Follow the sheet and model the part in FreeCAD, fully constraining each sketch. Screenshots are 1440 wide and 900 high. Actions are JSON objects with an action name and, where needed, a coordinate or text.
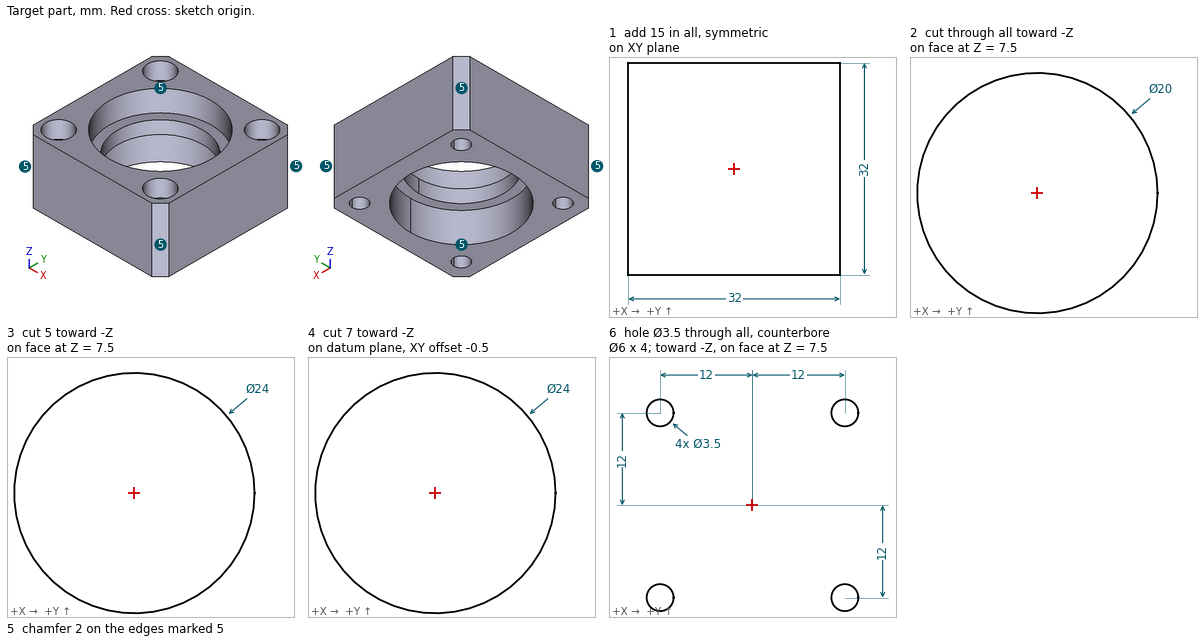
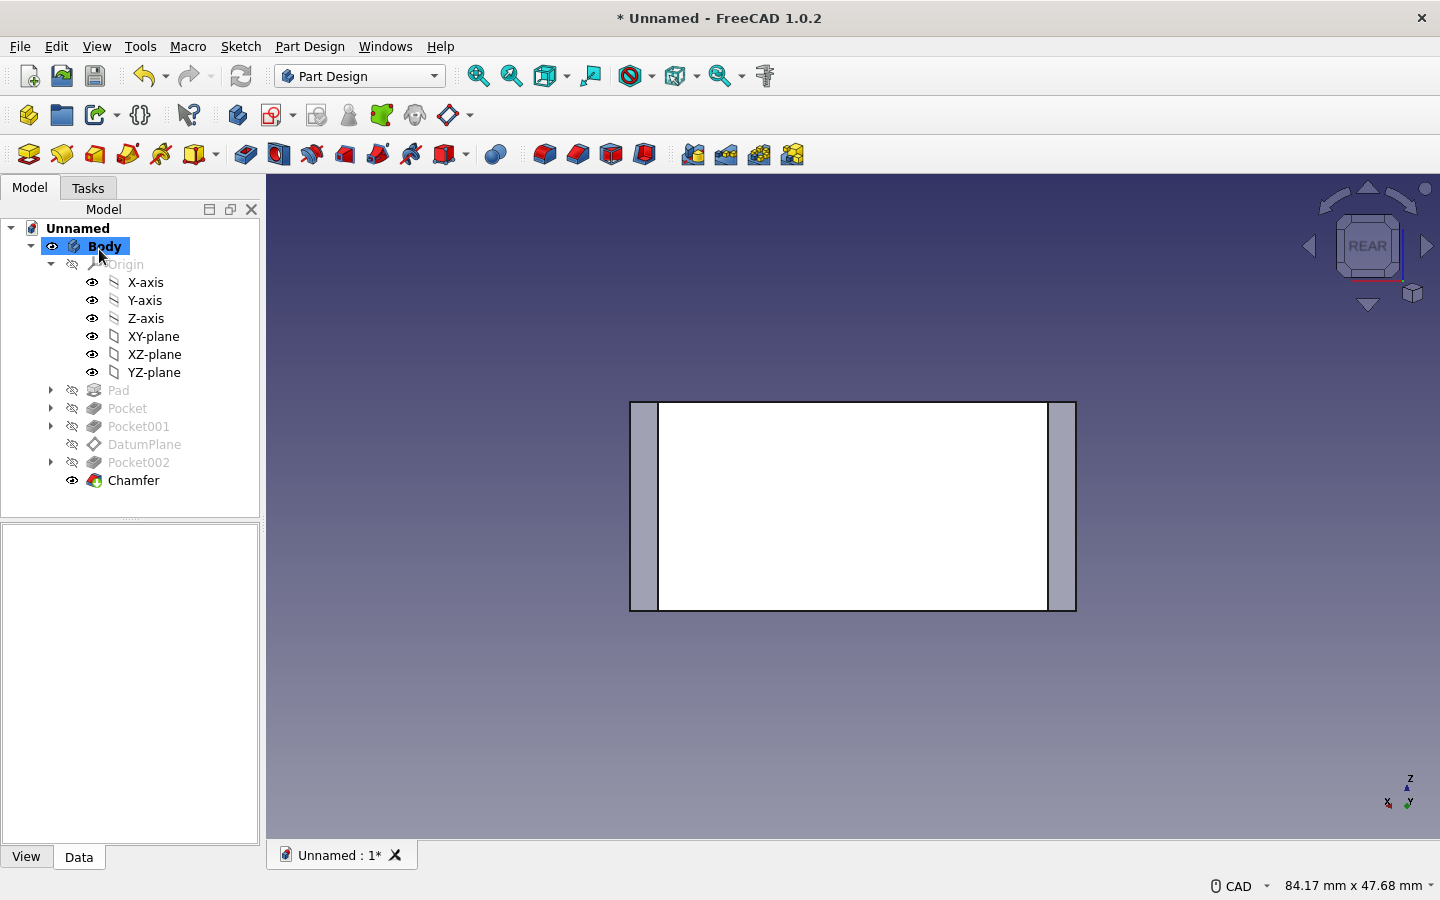
{"action": "key", "text": "v f"}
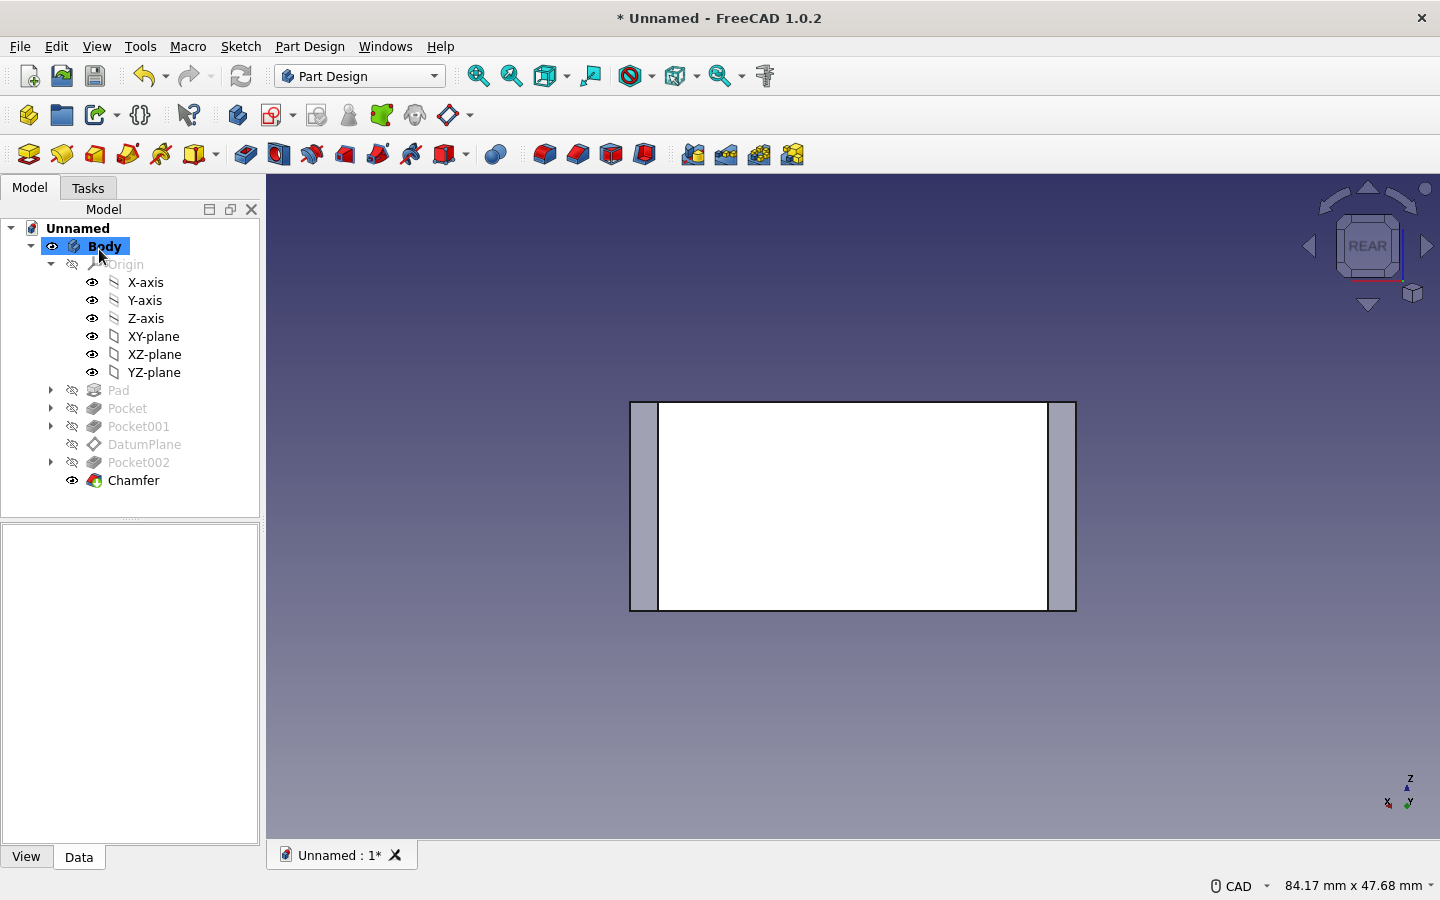
{"action": "key", "text": "0"}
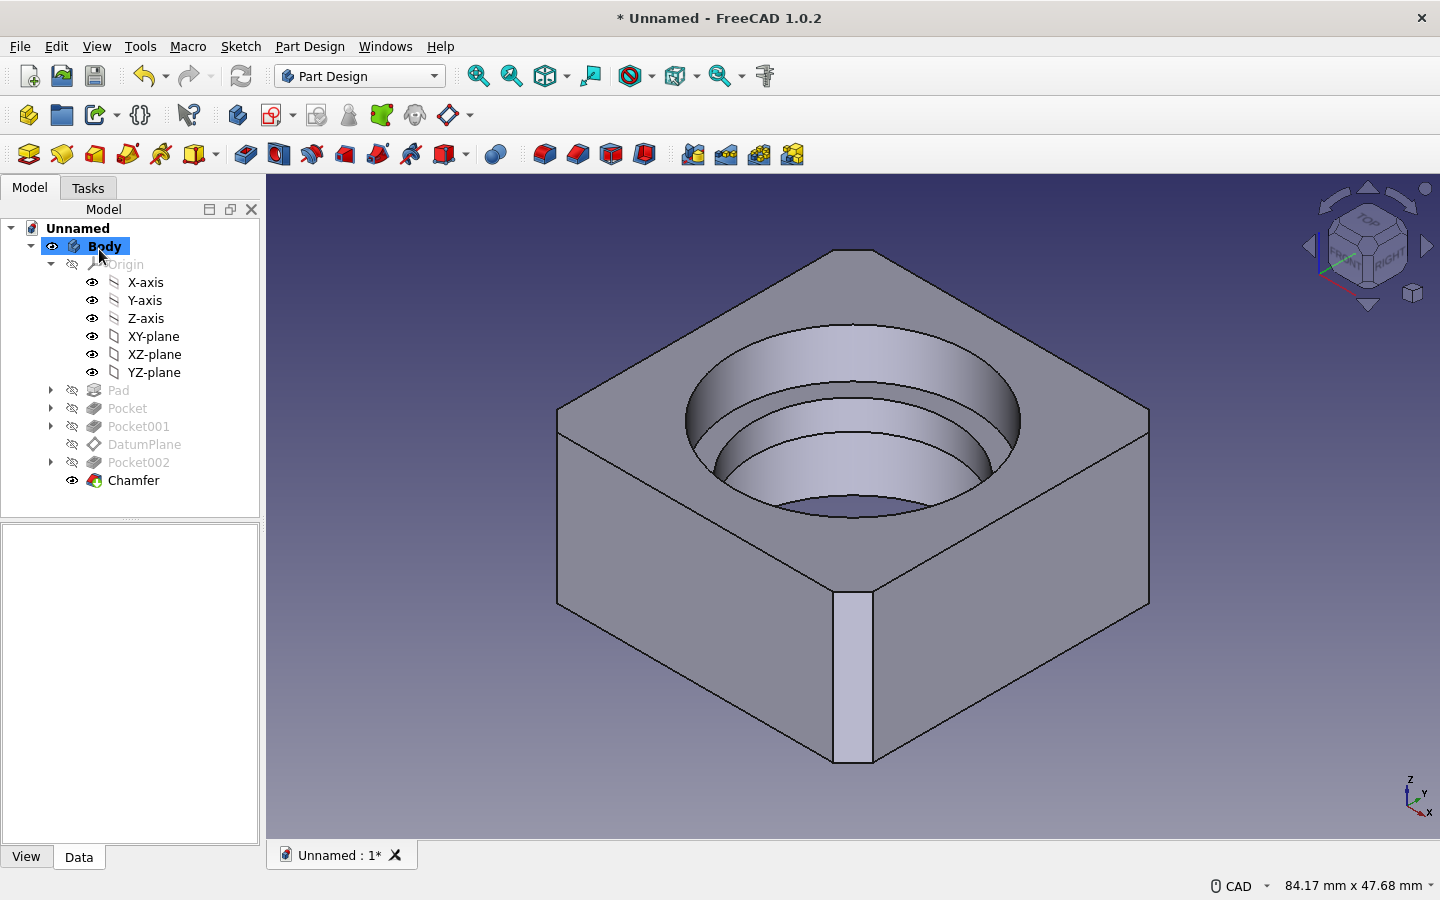
{"action": "left_click", "coordinate": [1078, 446]}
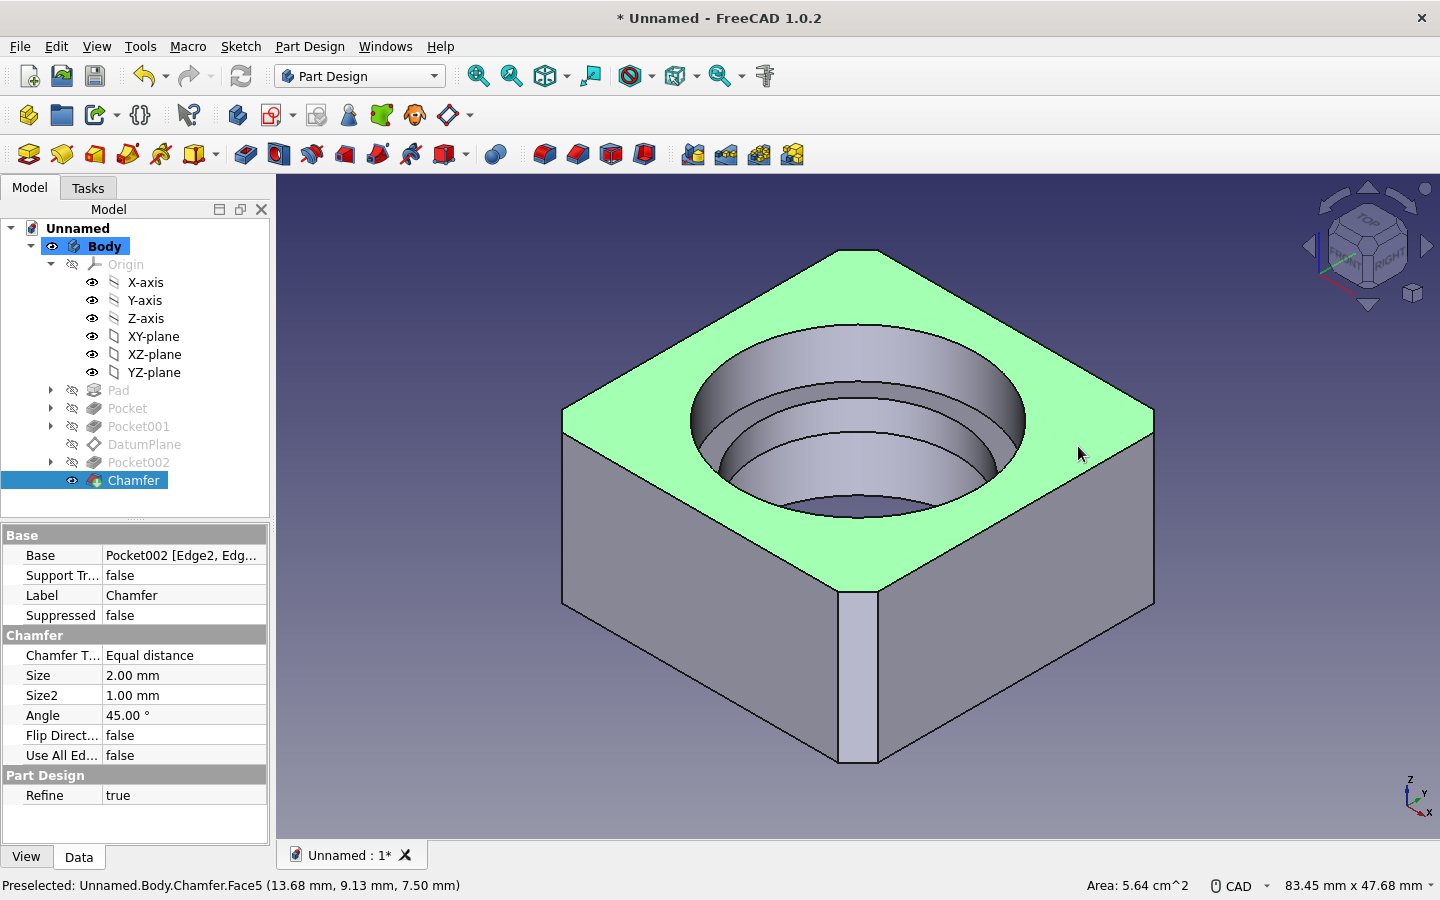
{"action": "left_click", "coordinate": [270, 116]}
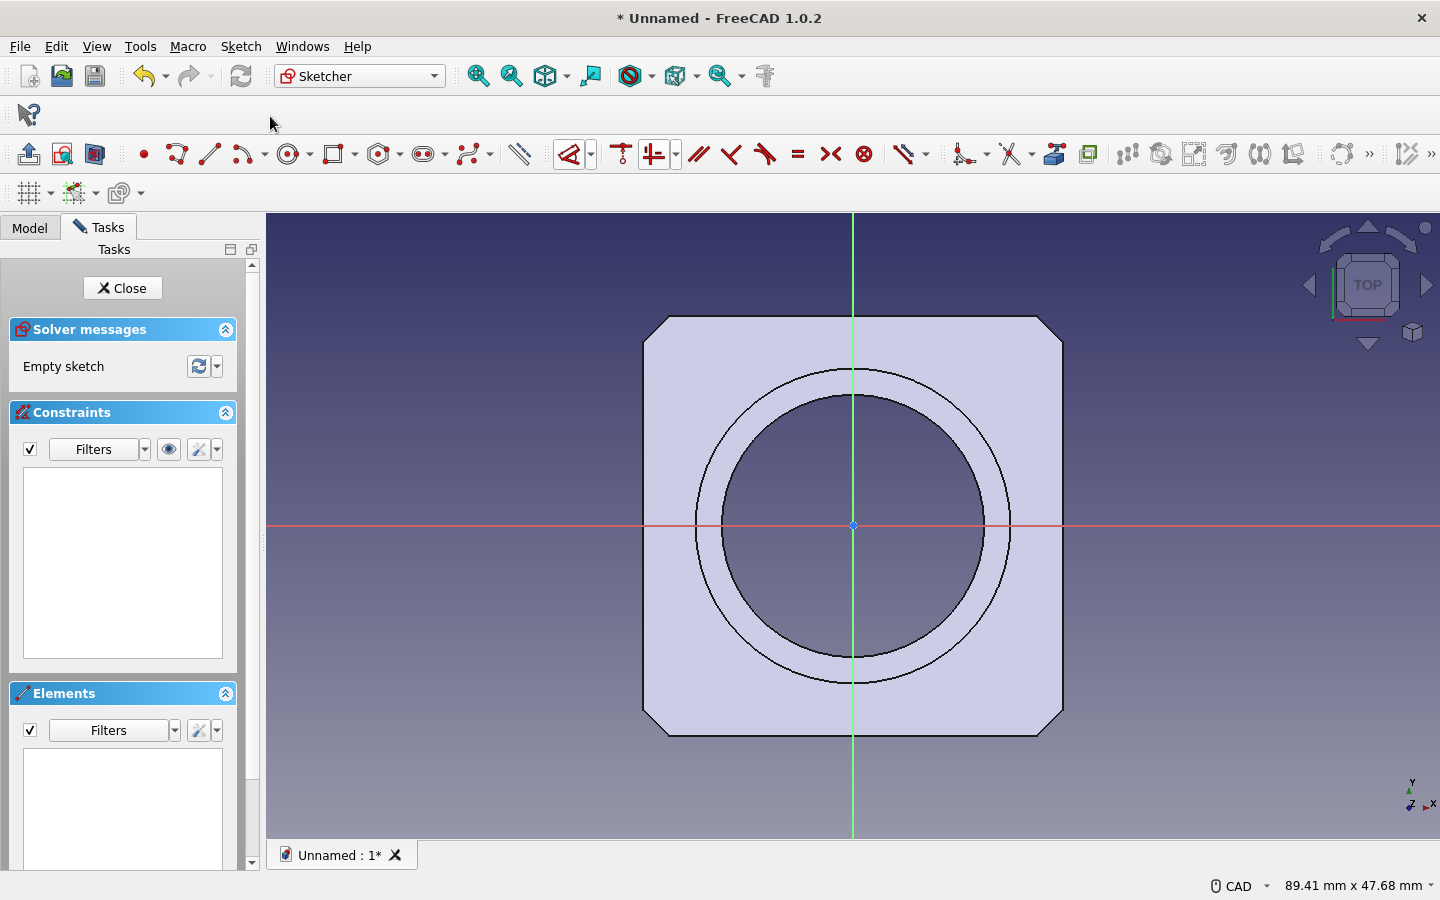
{"action": "left_click", "coordinate": [288, 154]}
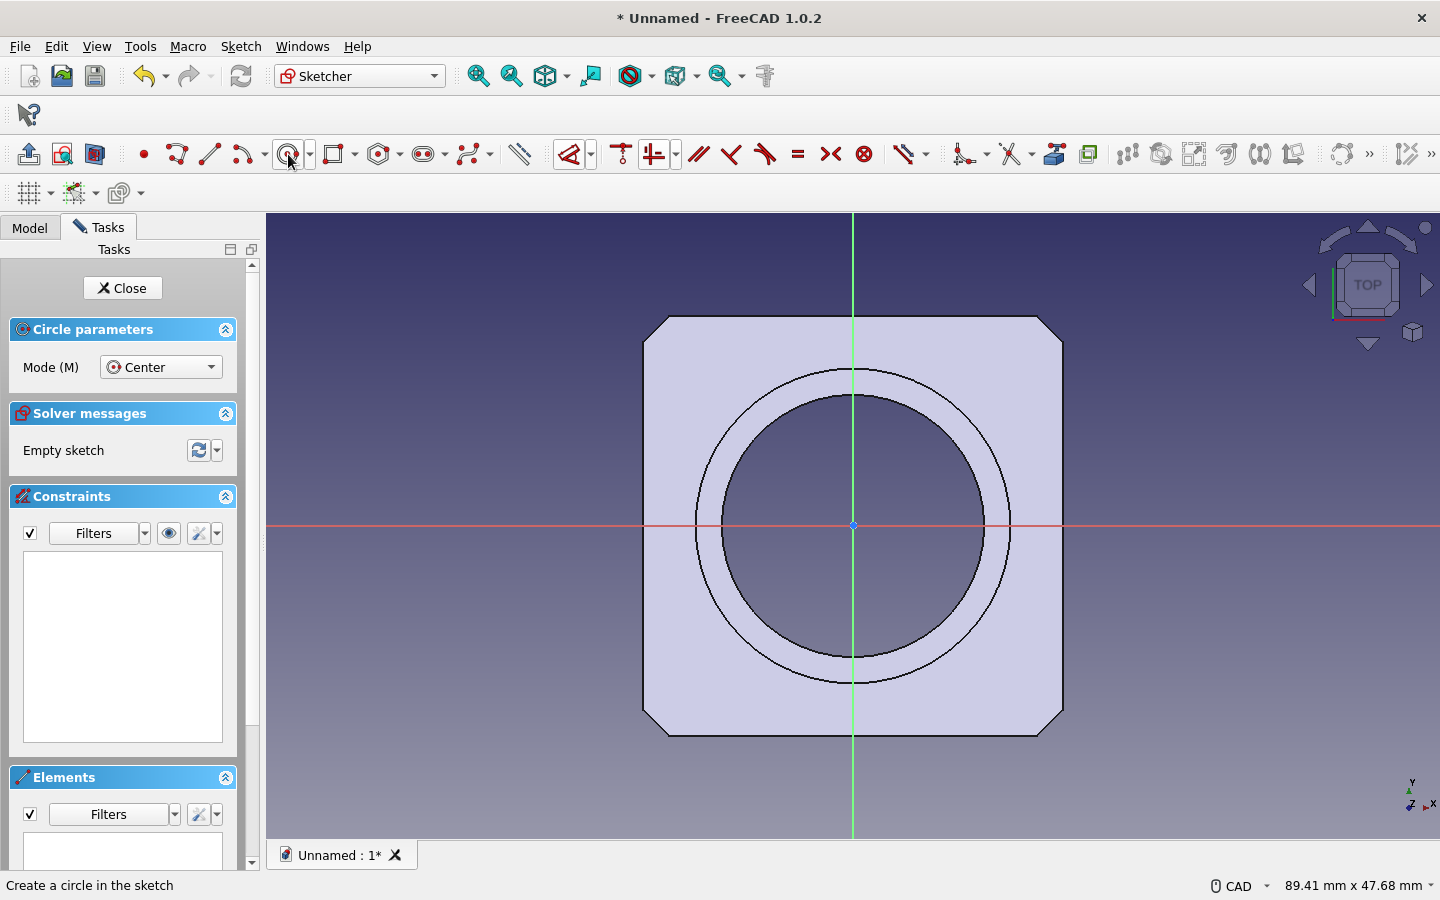
{"action": "left_click", "coordinate": [695, 368]}
{"action": "left_click", "coordinate": [712, 352]}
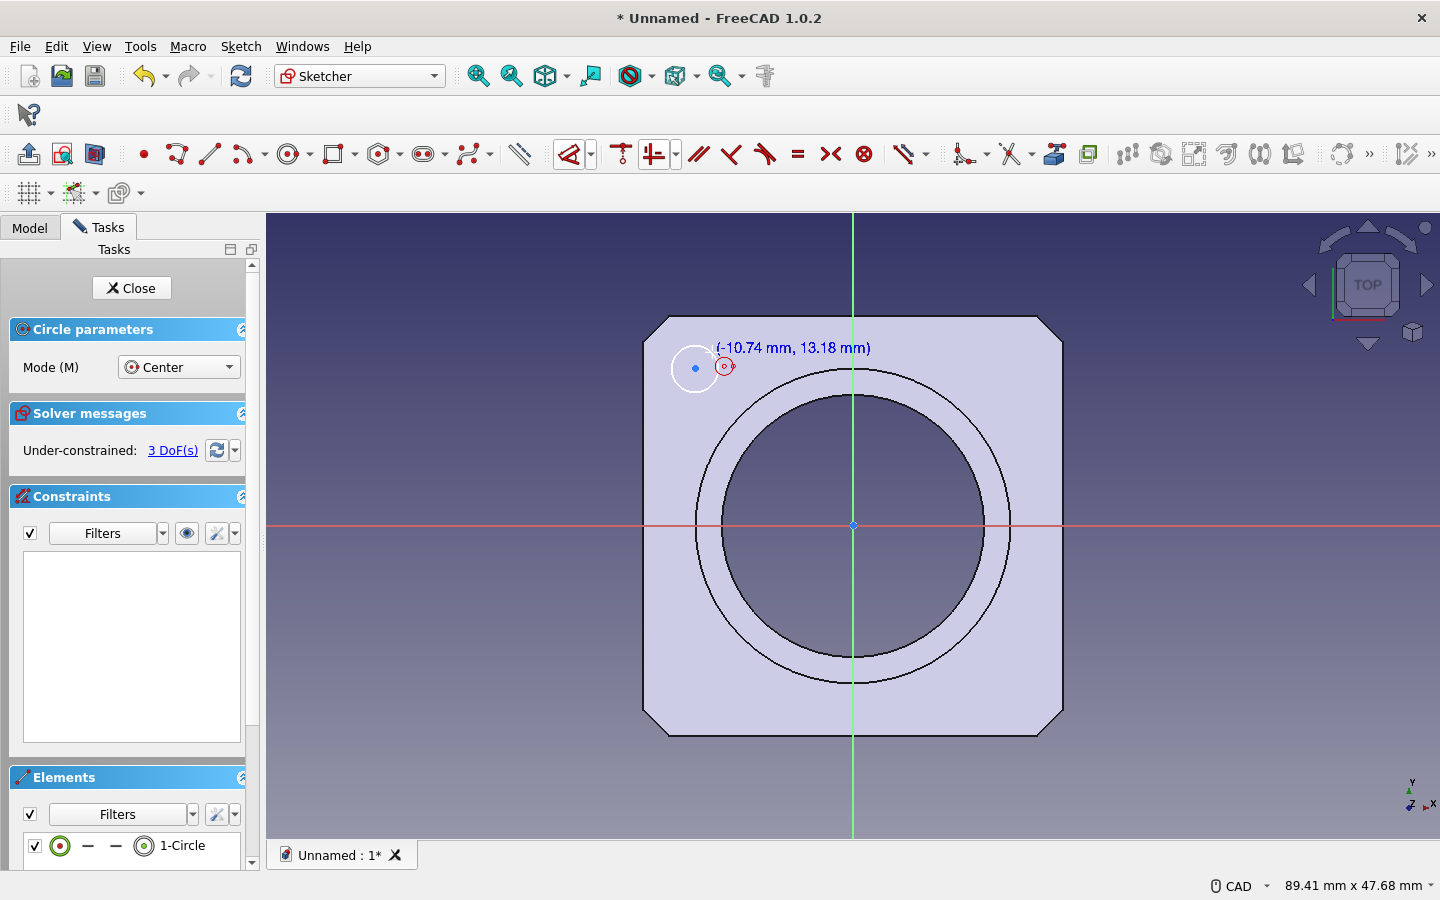
{"action": "left_click", "coordinate": [1011, 368]}
{"action": "left_click", "coordinate": [1027, 352]}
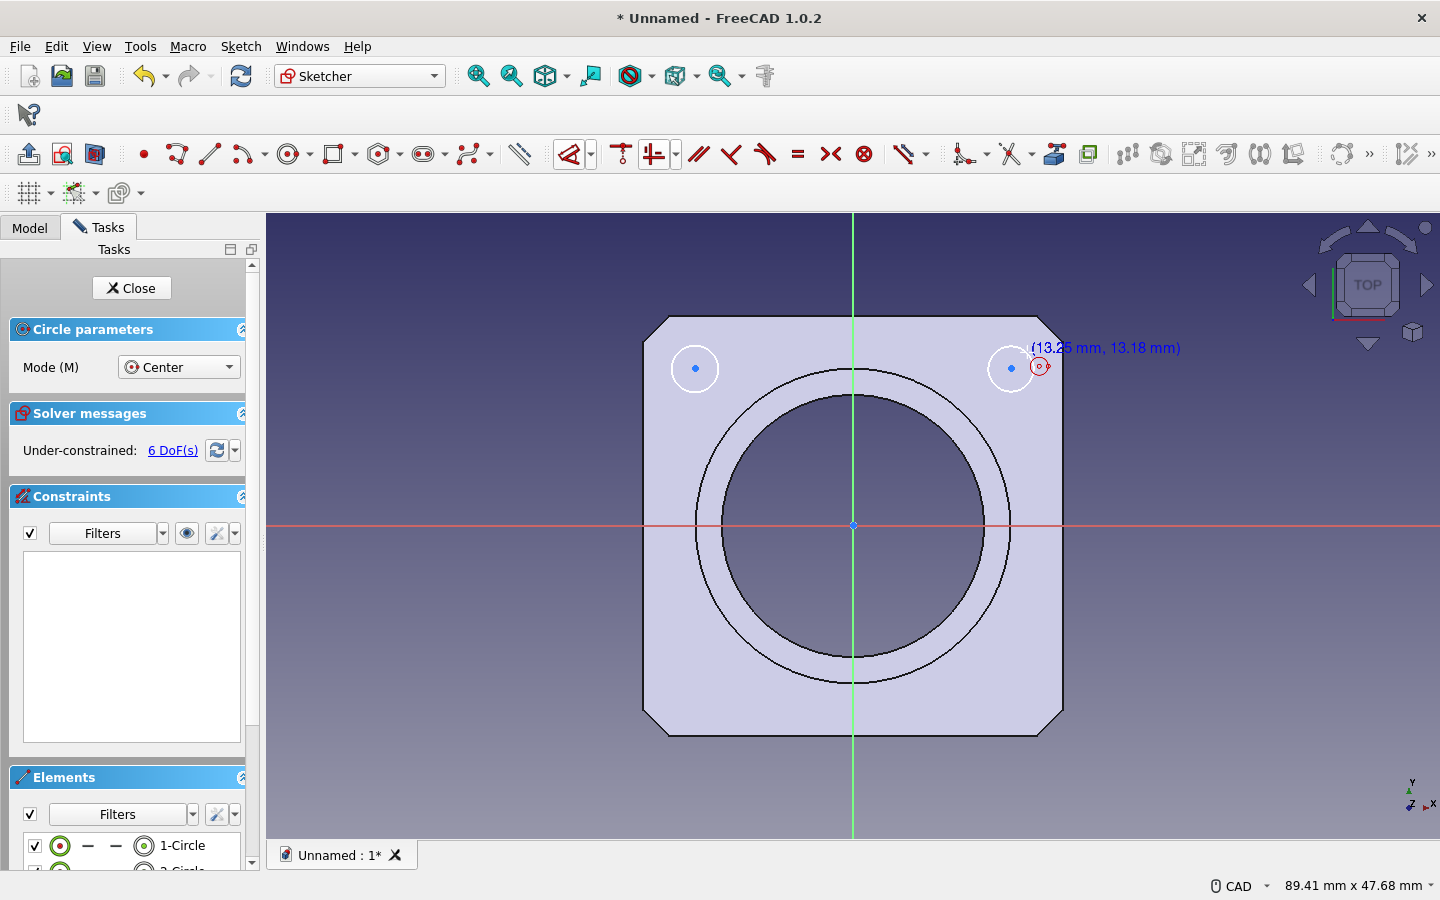
{"action": "left_click", "coordinate": [1011, 684]}
{"action": "left_click", "coordinate": [1027, 667]}